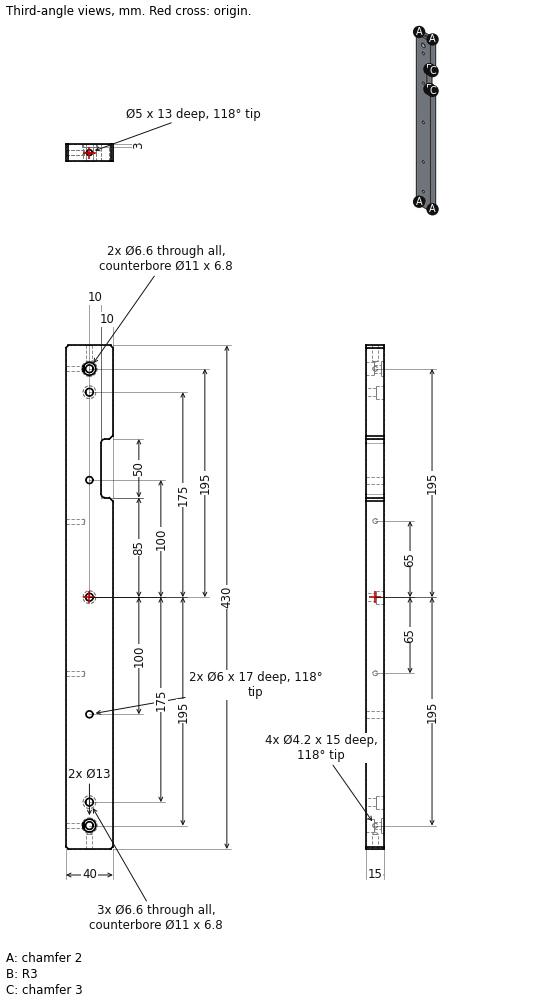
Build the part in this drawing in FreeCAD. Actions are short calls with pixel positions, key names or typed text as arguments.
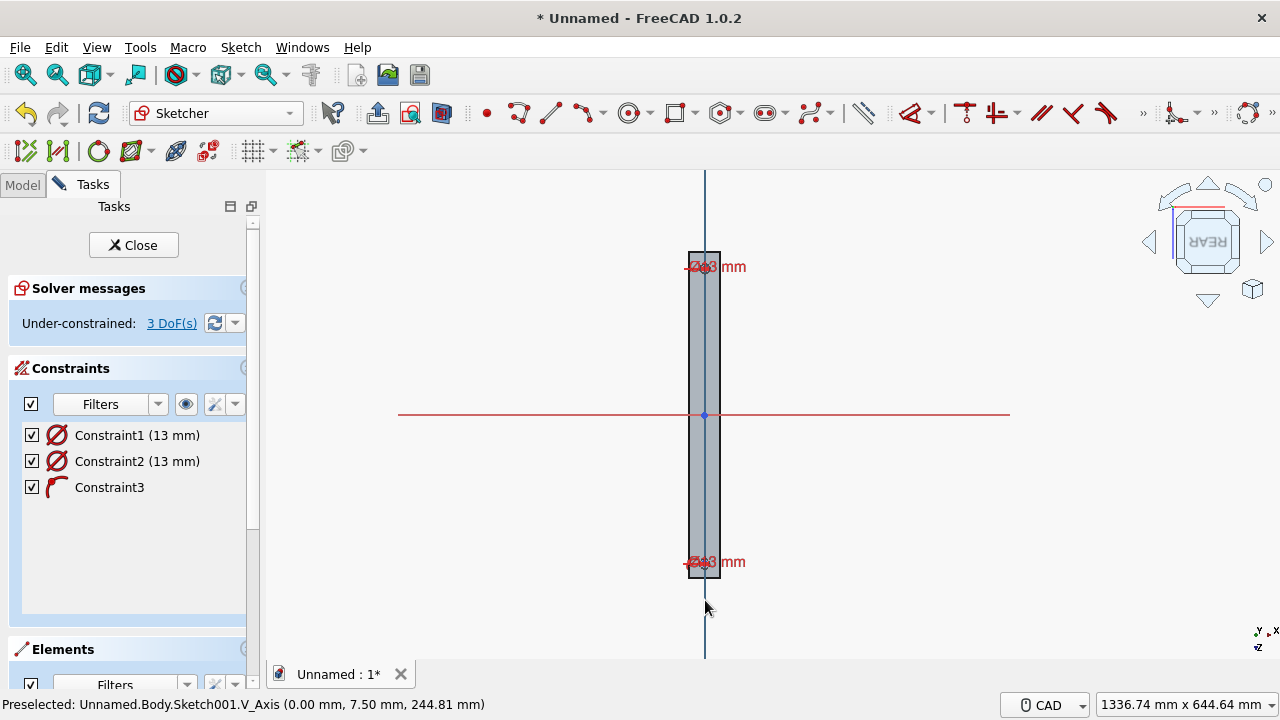
click(966, 114)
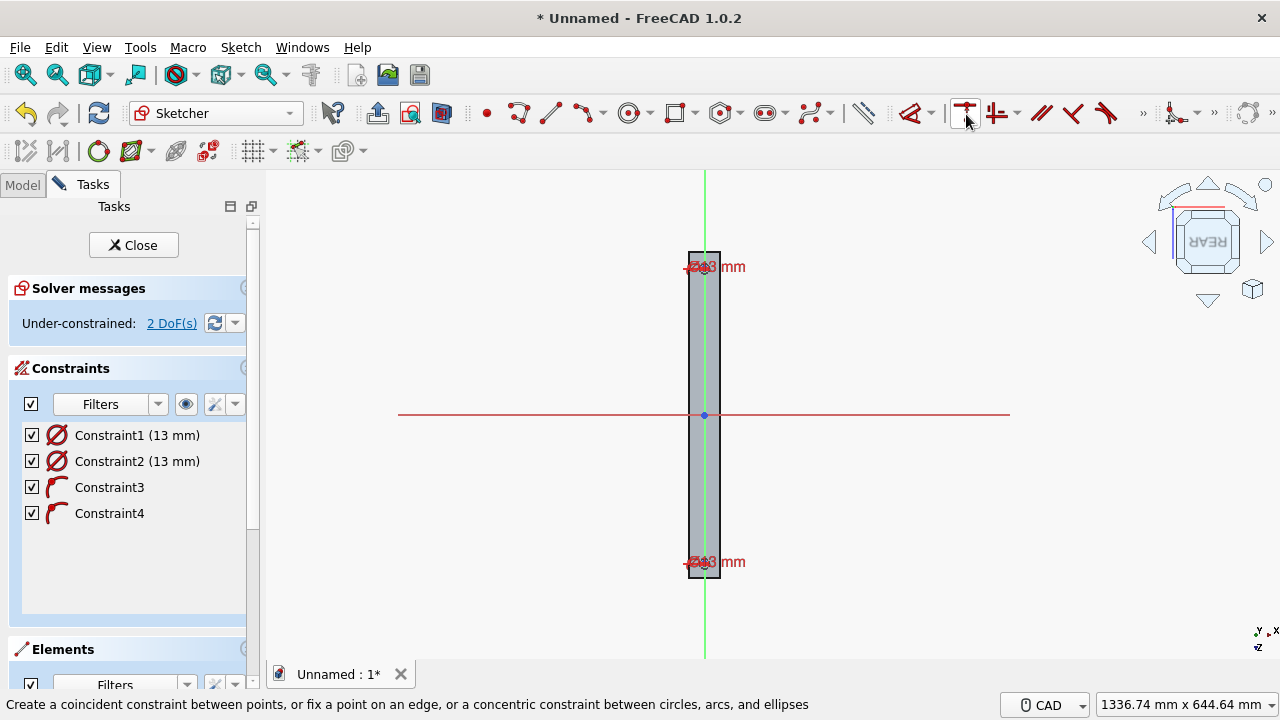
click(910, 114)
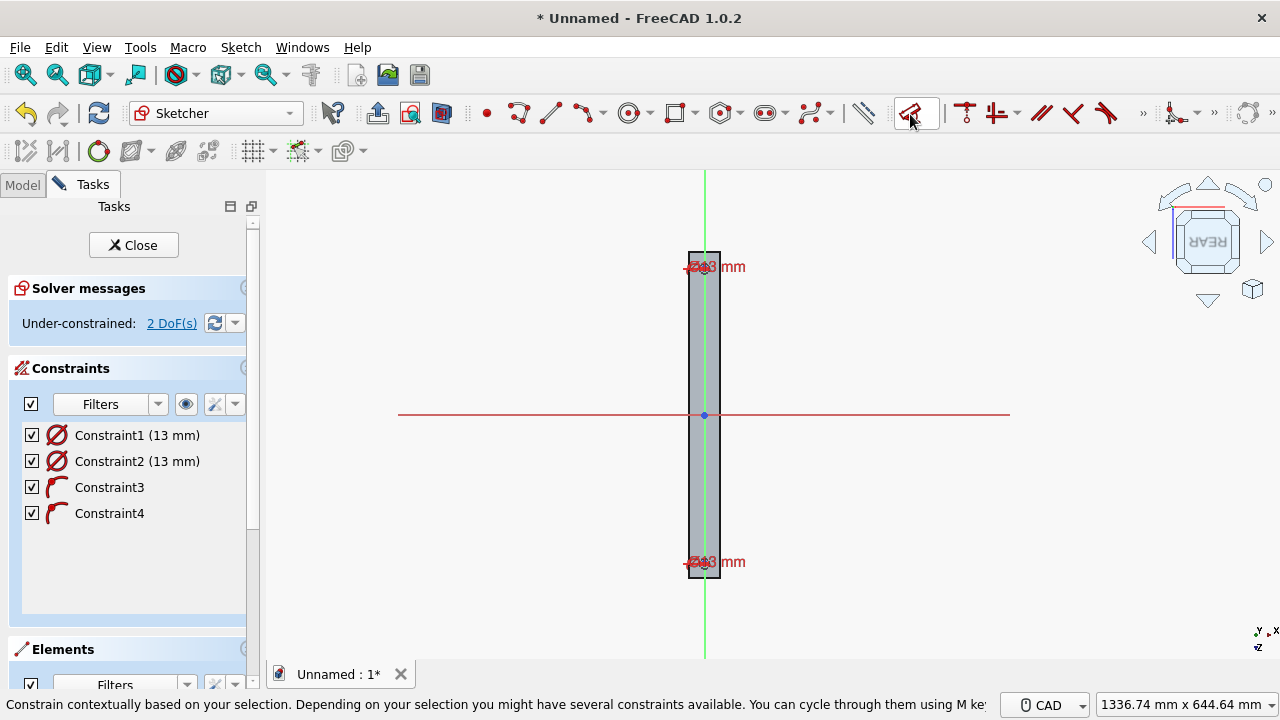
click(705, 269)
click(739, 342)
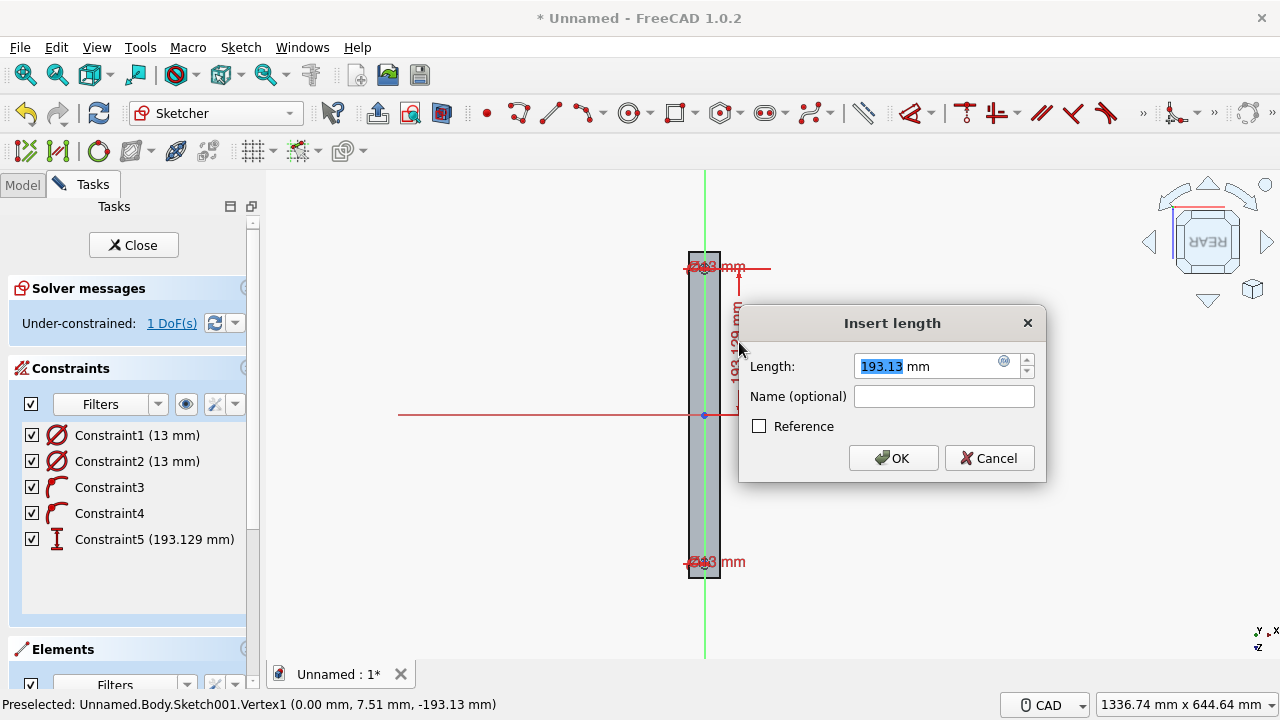
text(195)
key(Return)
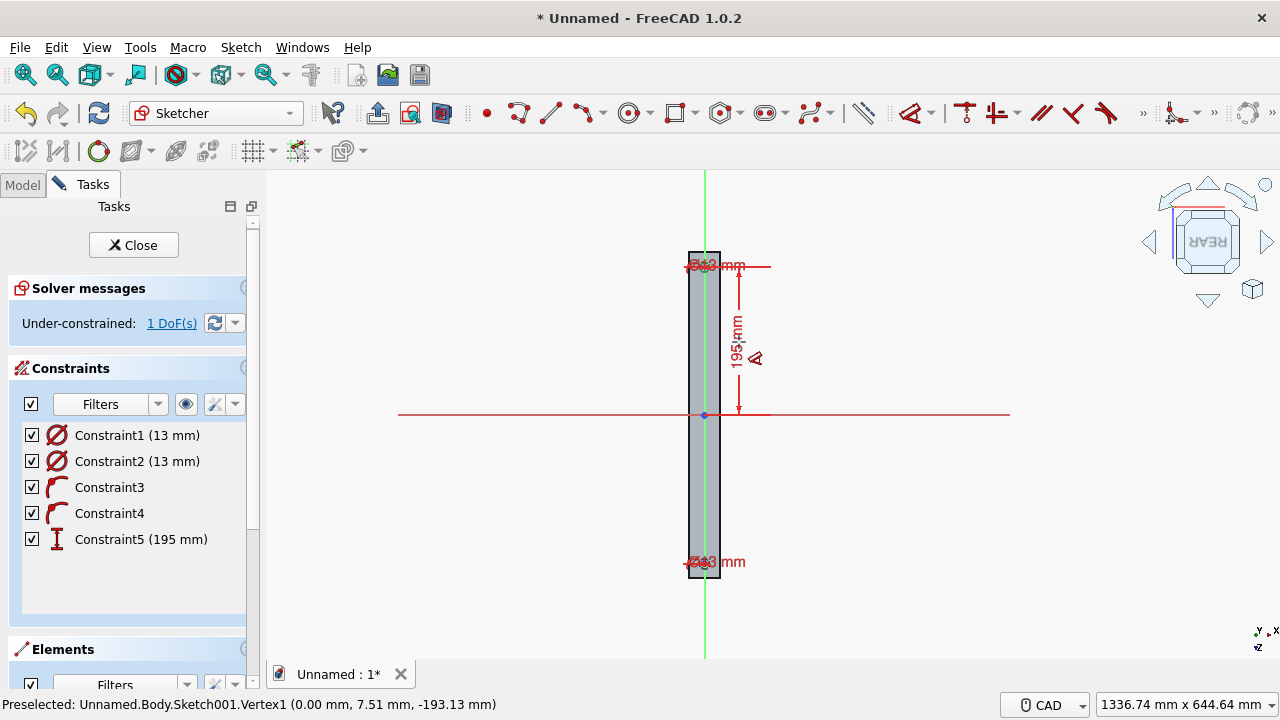
click(705, 564)
click(739, 490)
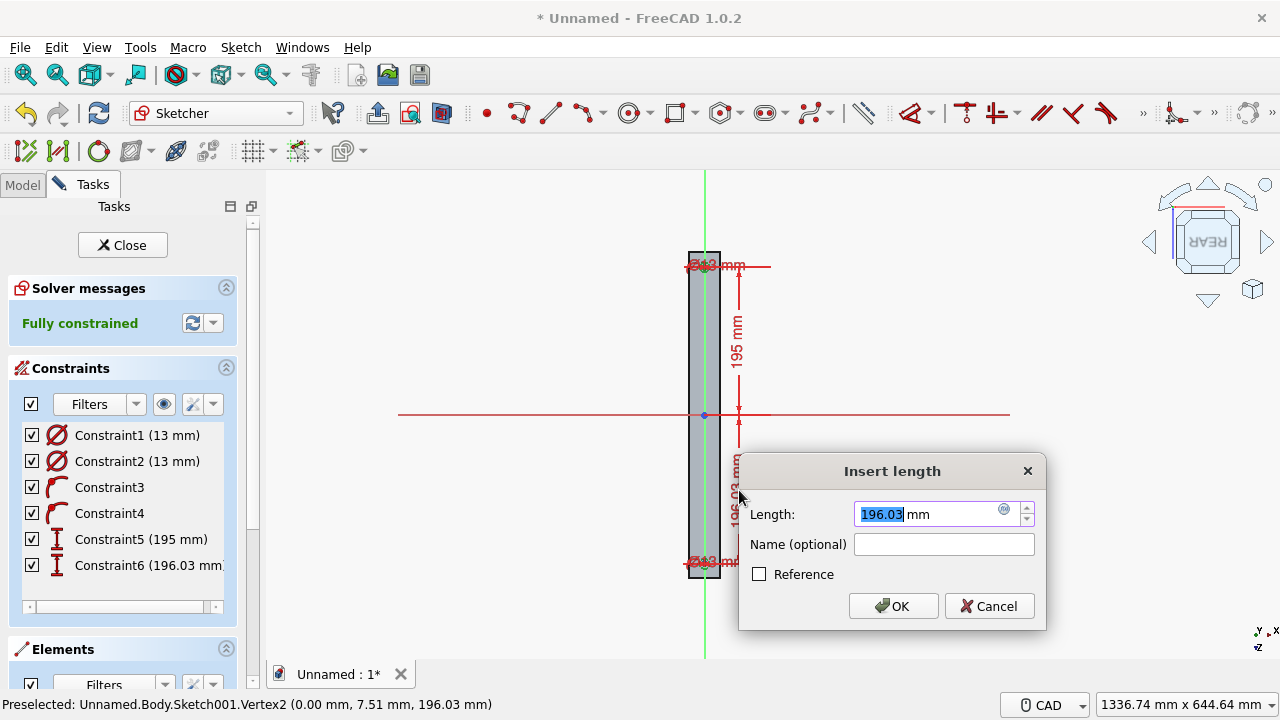
text(195)
key(Return)
key(Escape)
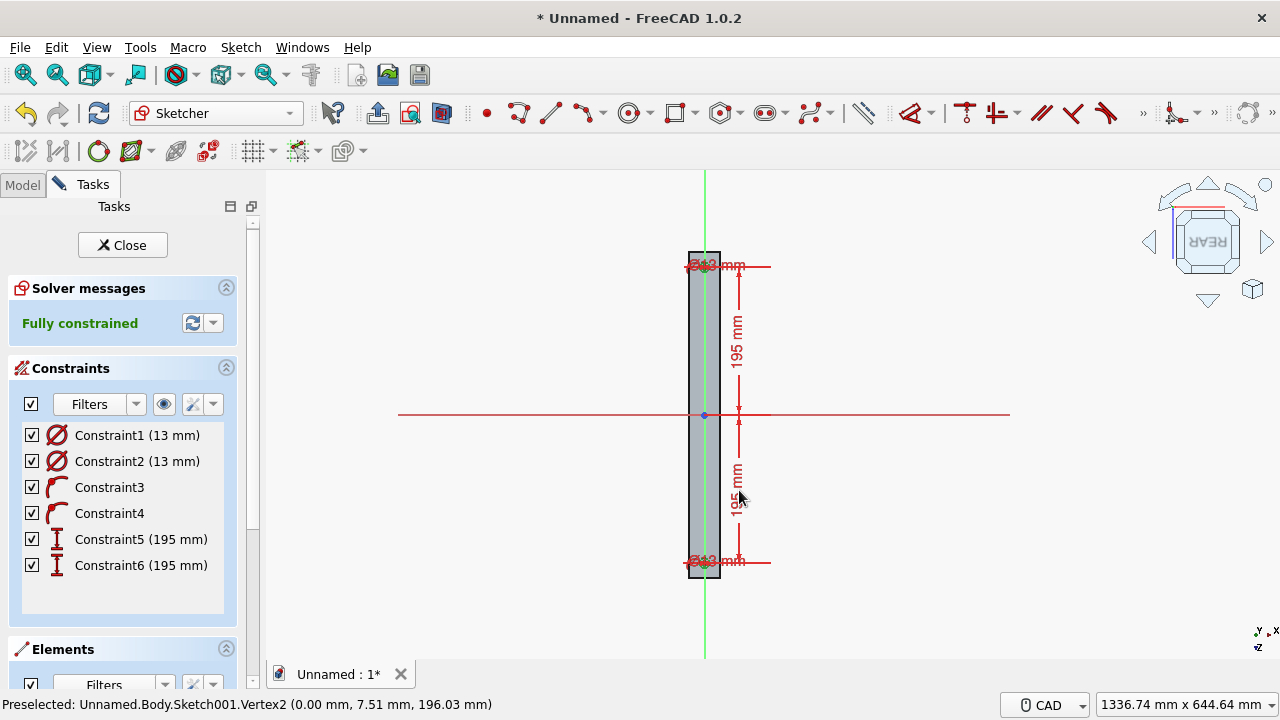
click(123, 245)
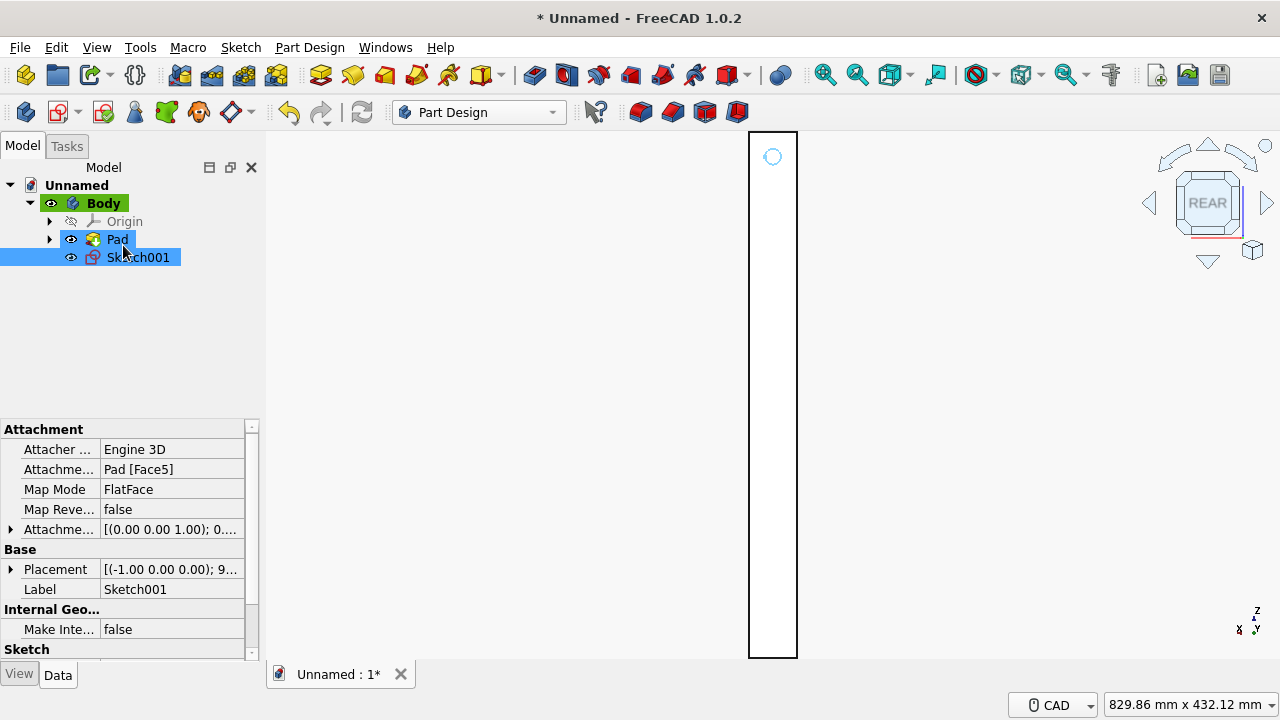
click(536, 76)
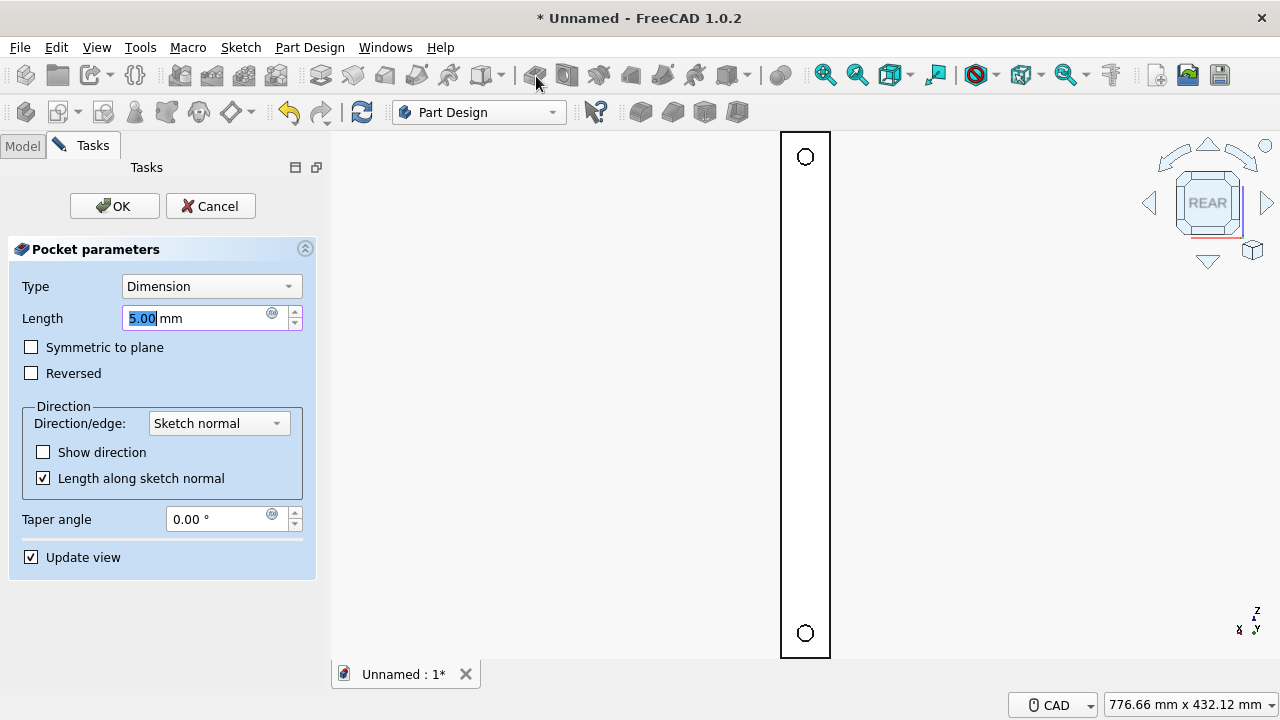
text(3)
key(Tab)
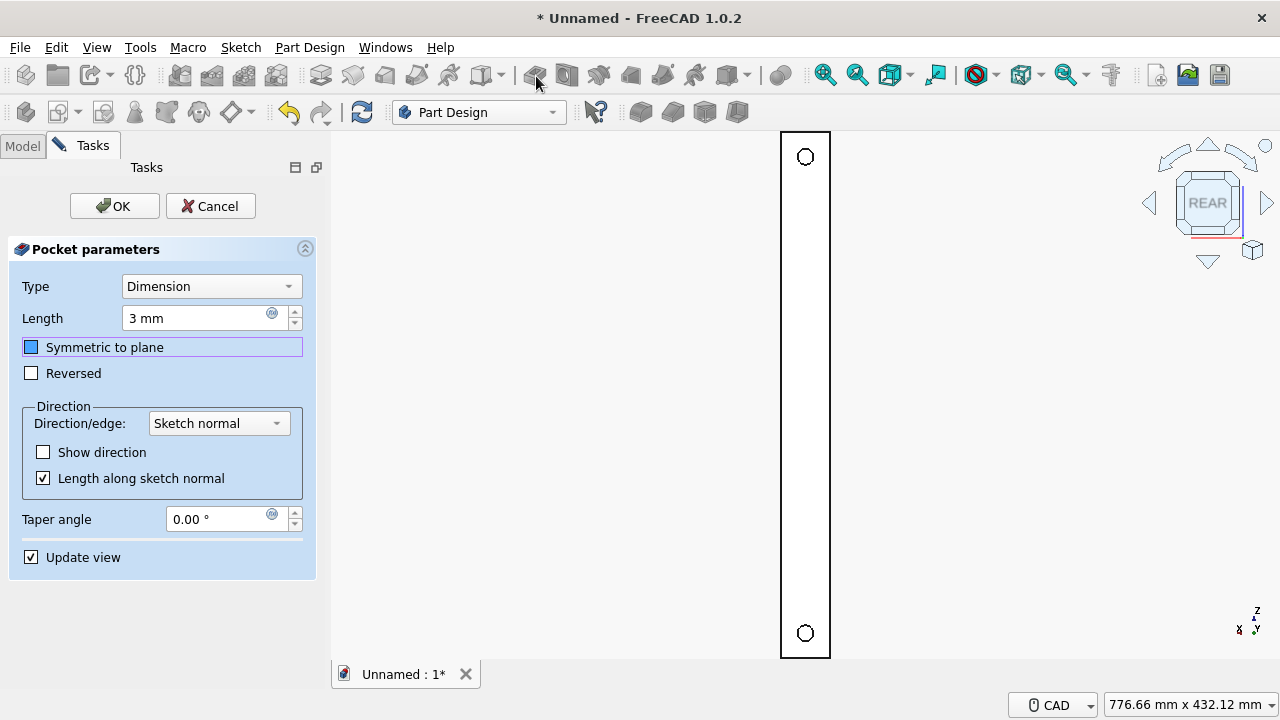
click(115, 206)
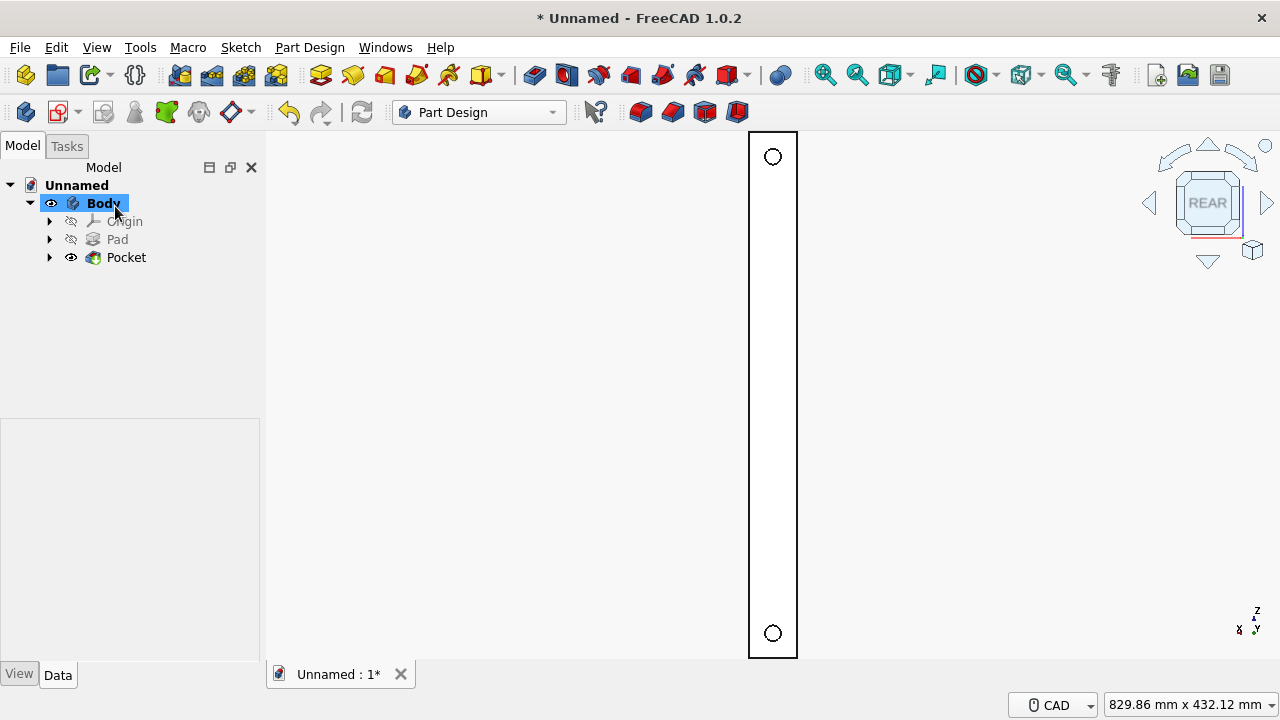
key(0)